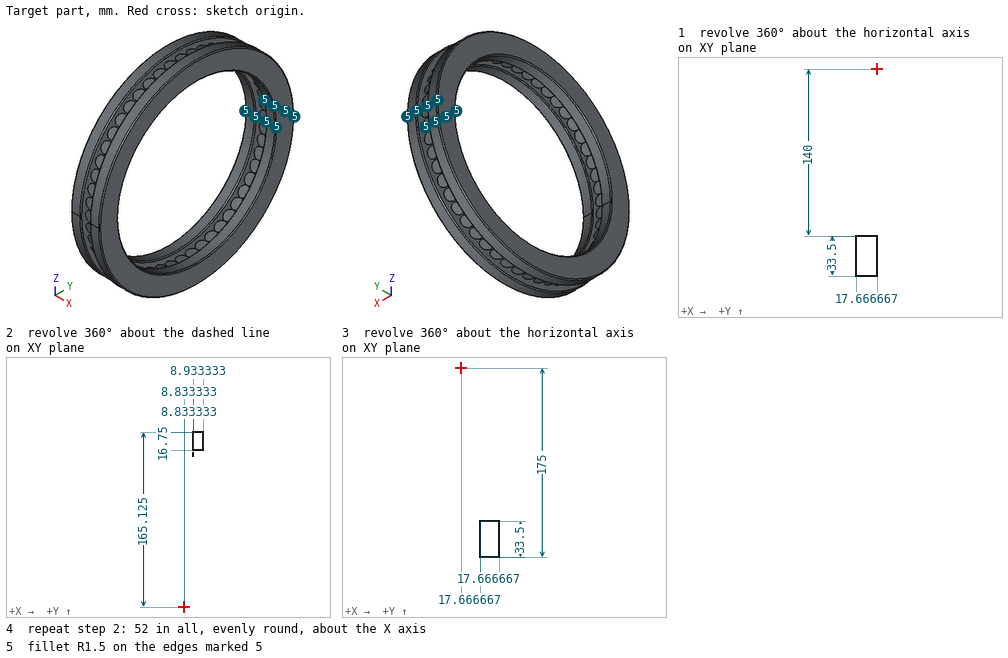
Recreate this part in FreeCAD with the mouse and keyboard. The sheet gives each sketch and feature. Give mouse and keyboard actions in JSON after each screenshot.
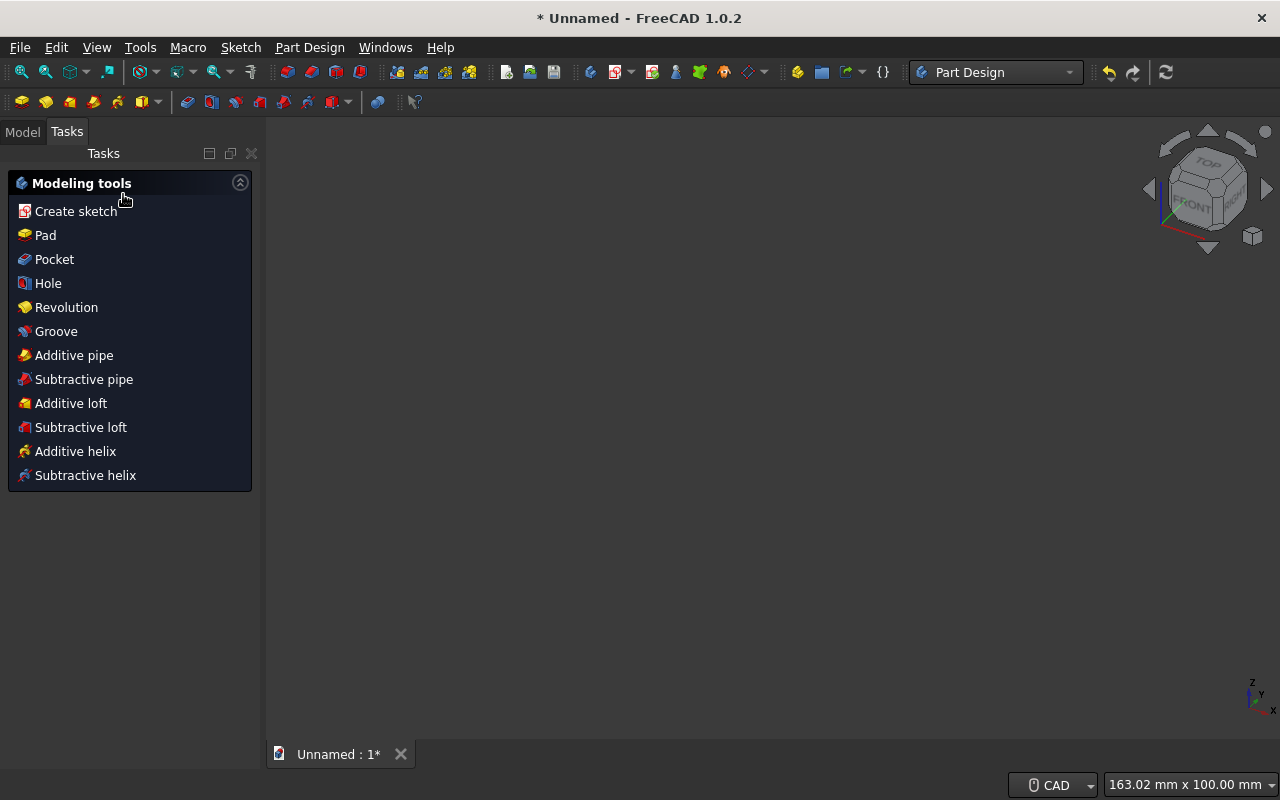
{"action": "left_click", "coordinate": [46, 102]}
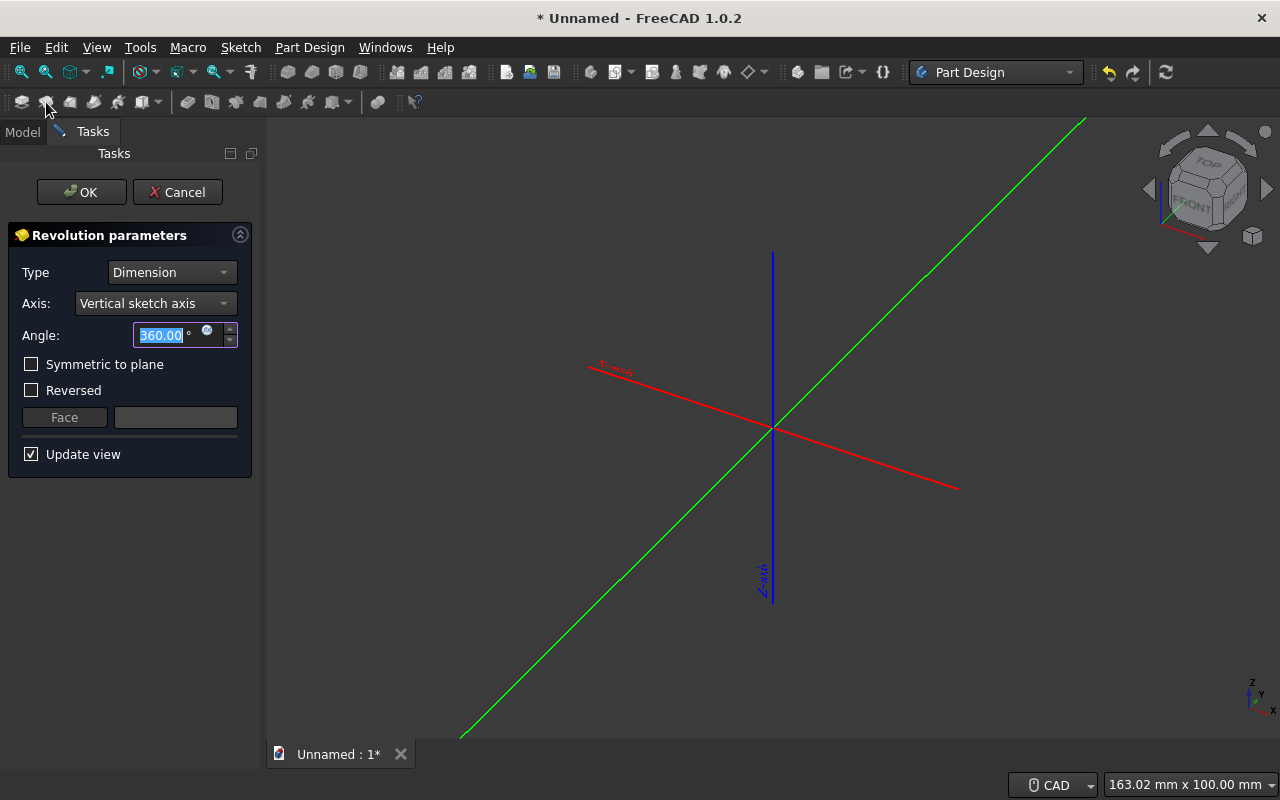
{"action": "left_click", "coordinate": [156, 304]}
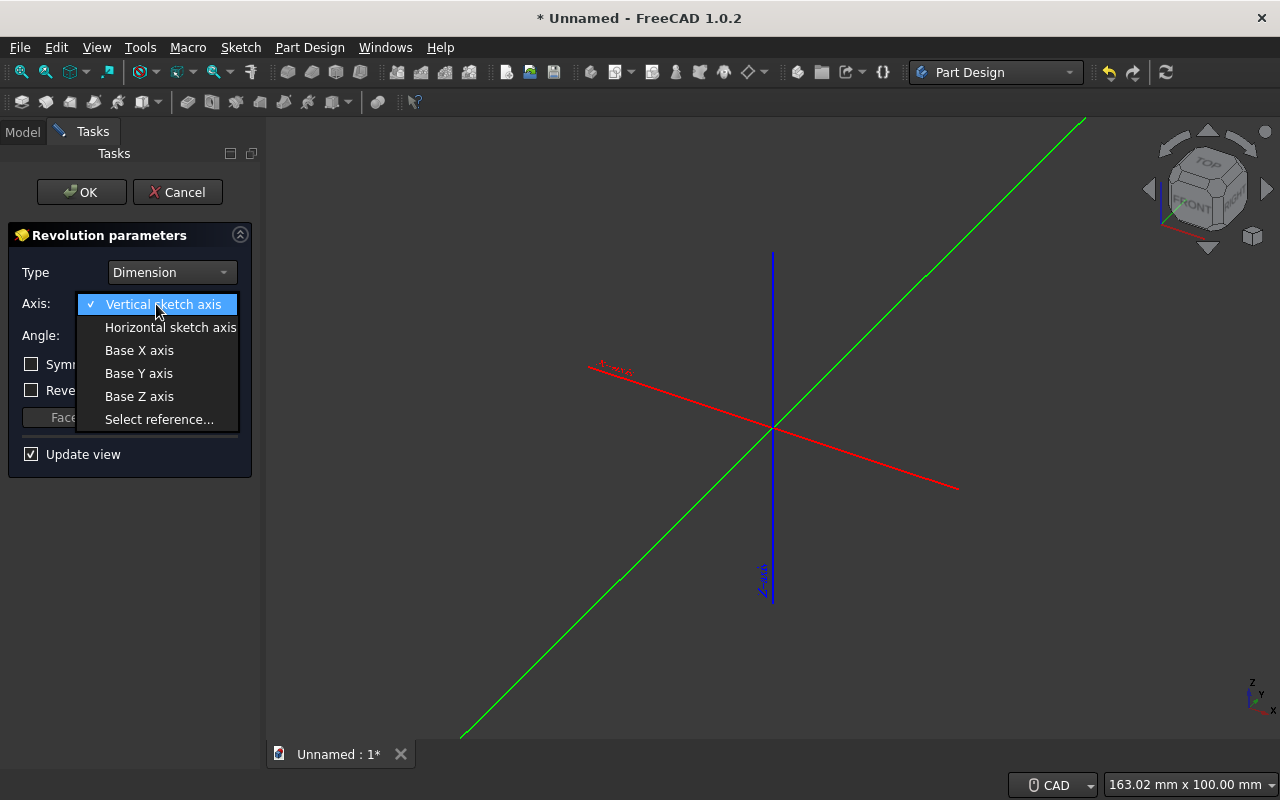
{"action": "left_click", "coordinate": [156, 328]}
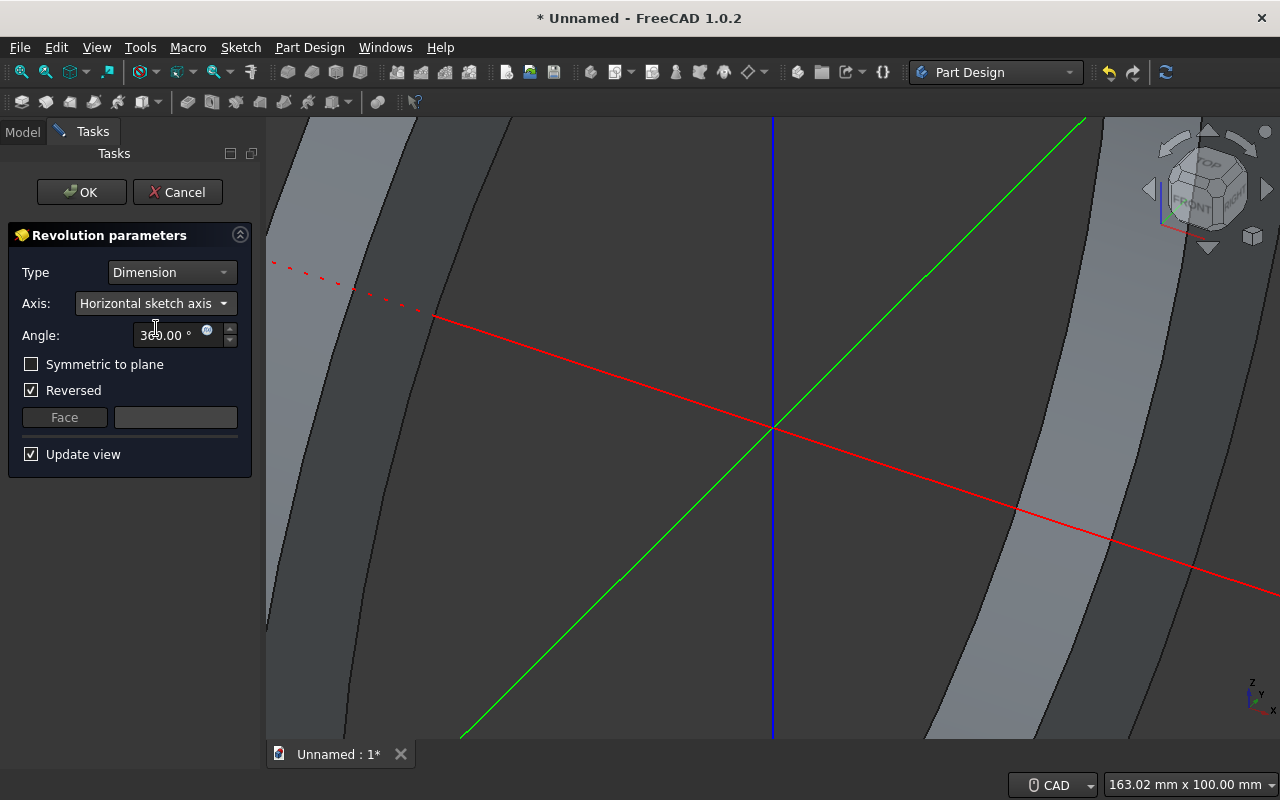
{"action": "left_click", "coordinate": [82, 192]}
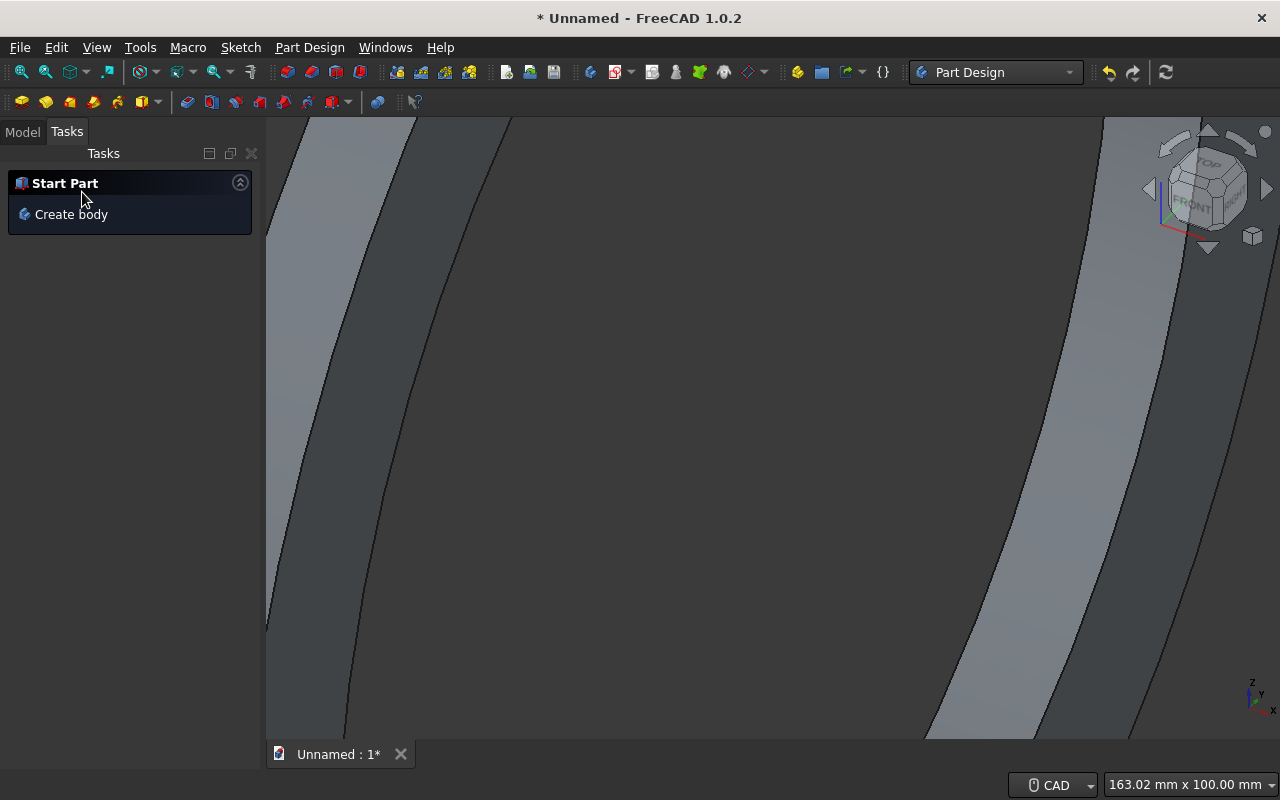
{"action": "left_click", "coordinate": [22, 72]}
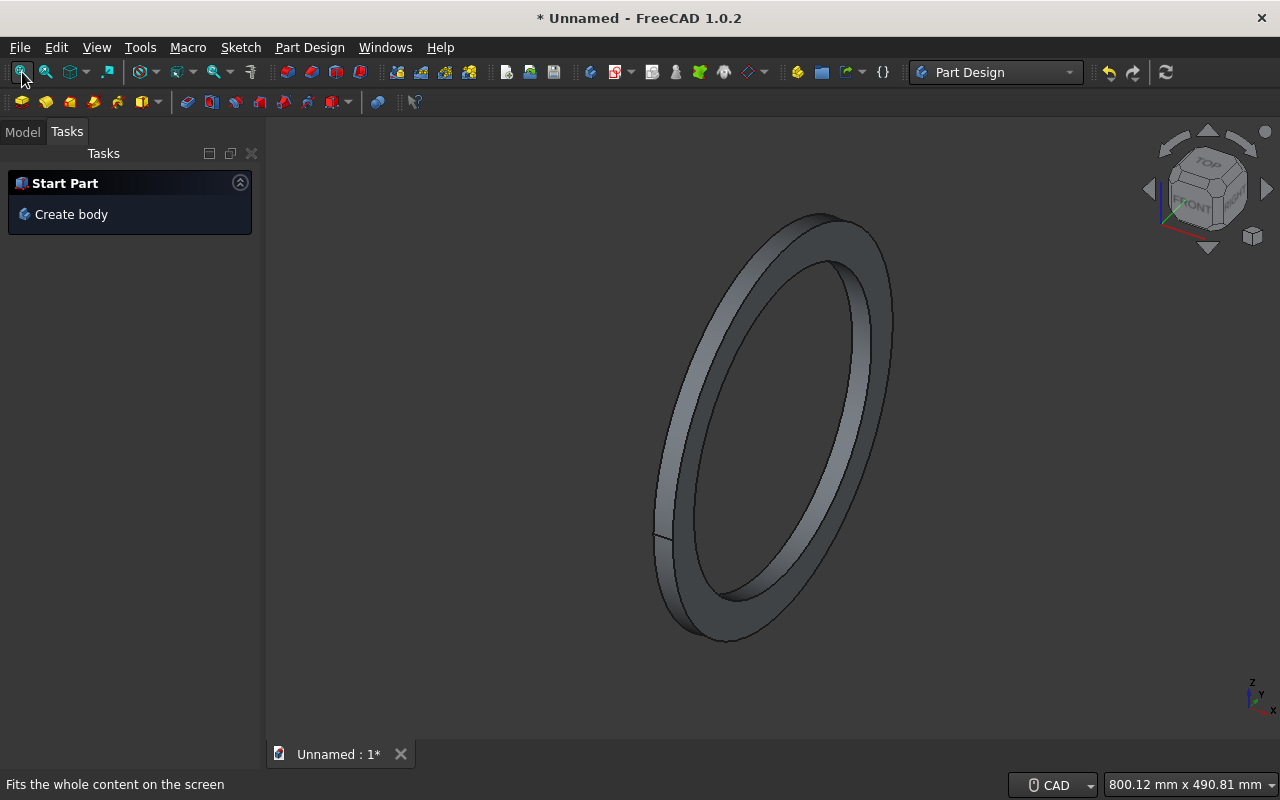
{"action": "left_click", "coordinate": [616, 72]}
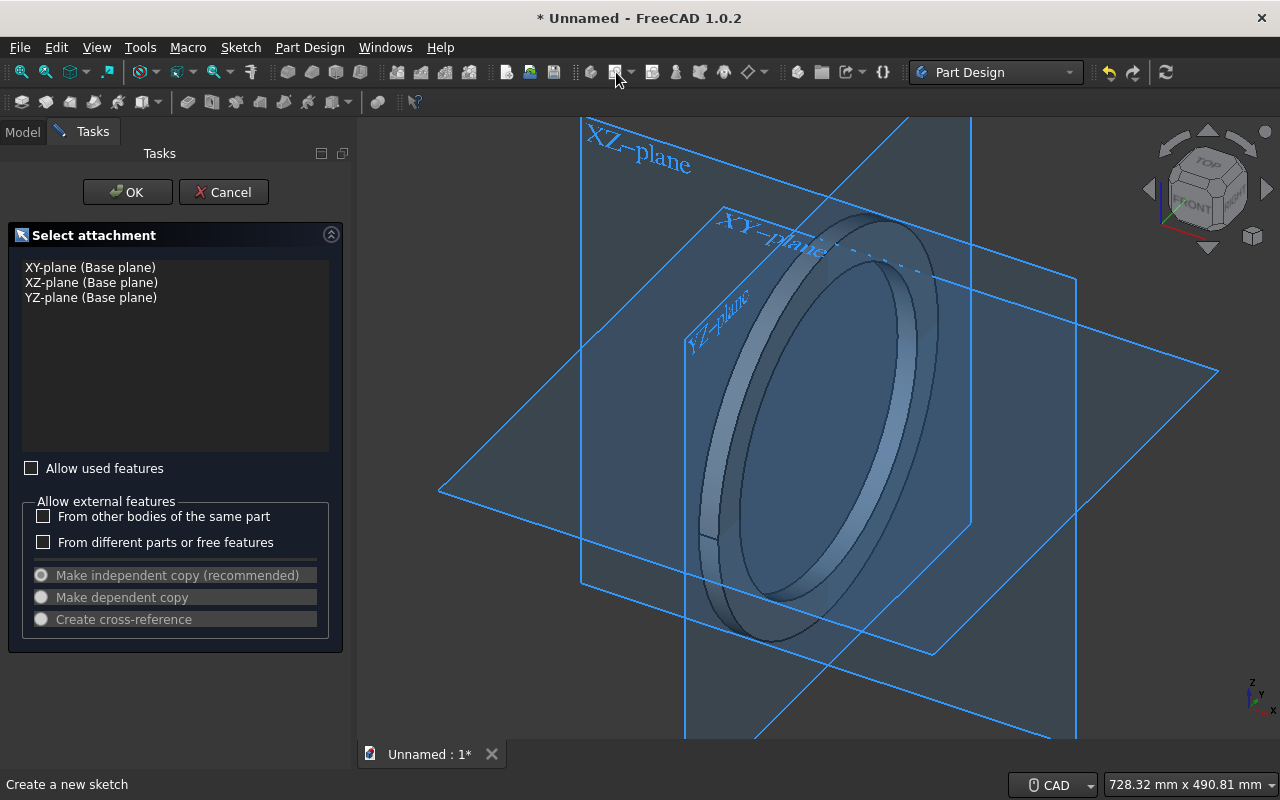
{"action": "left_click", "coordinate": [82, 268]}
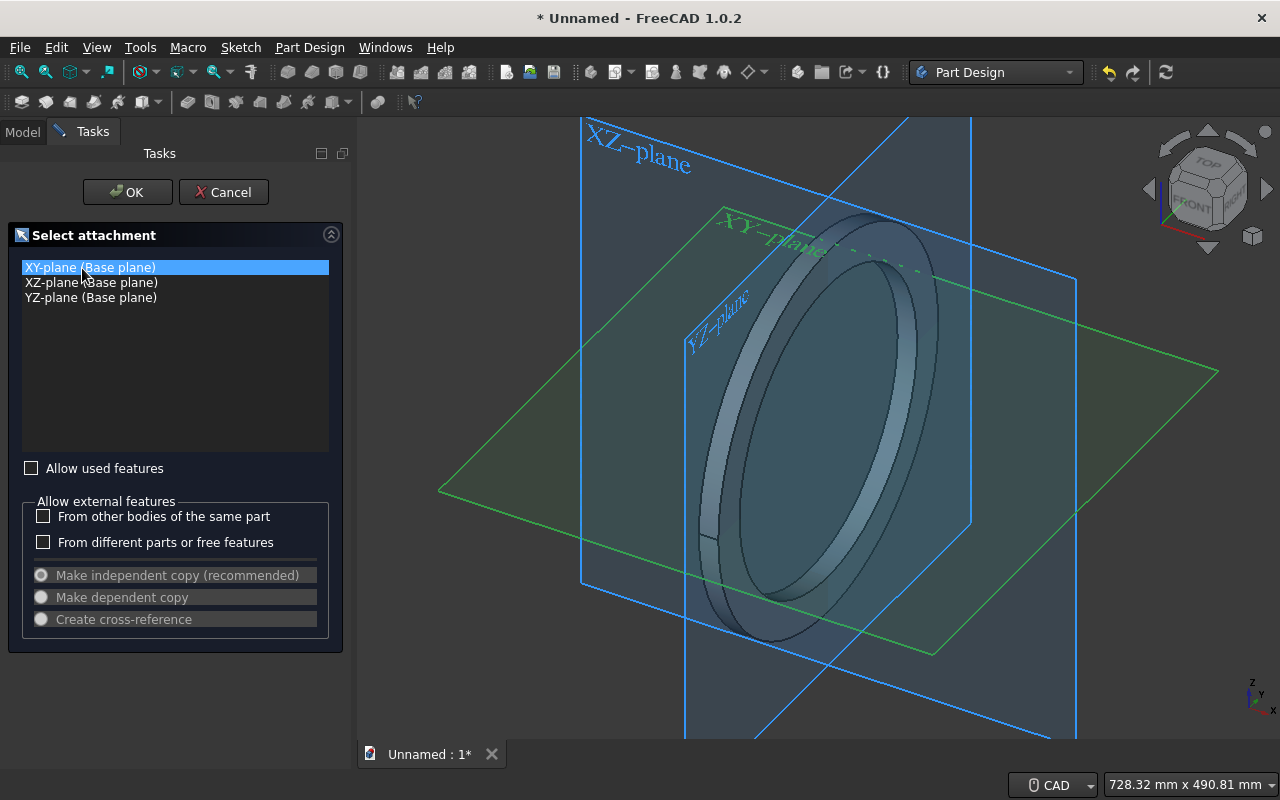
{"action": "left_click", "coordinate": [128, 192]}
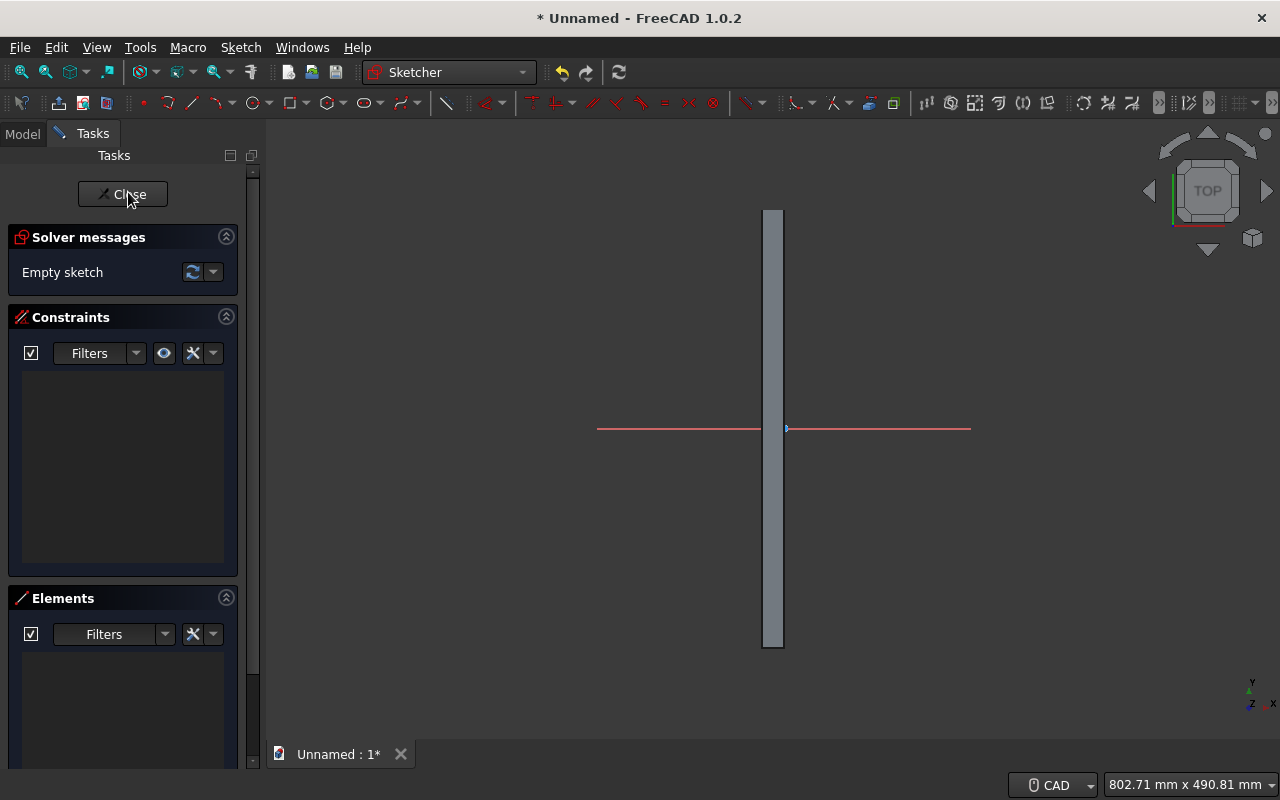
{"action": "key", "text": "q s"}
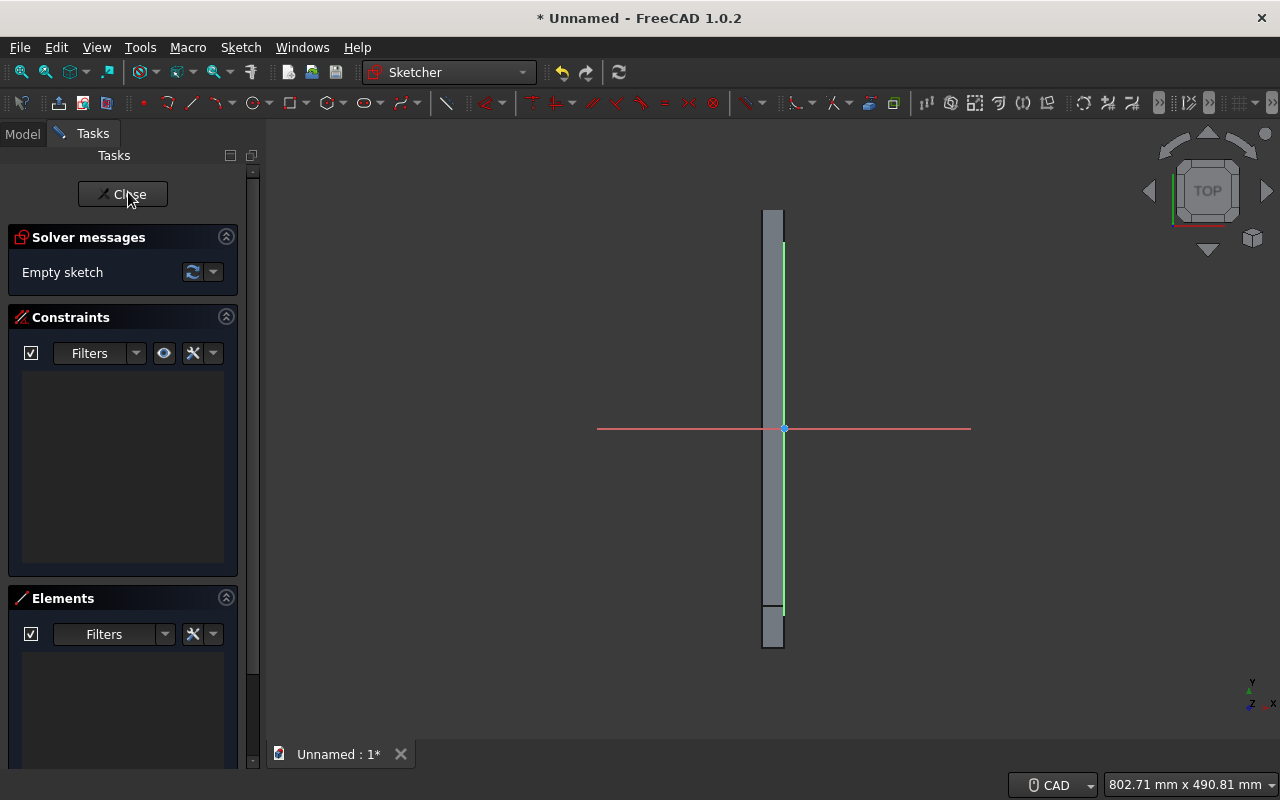
{"action": "scroll", "coordinate": [809, 220], "scroll_direction": "up", "scroll_amount": 13}